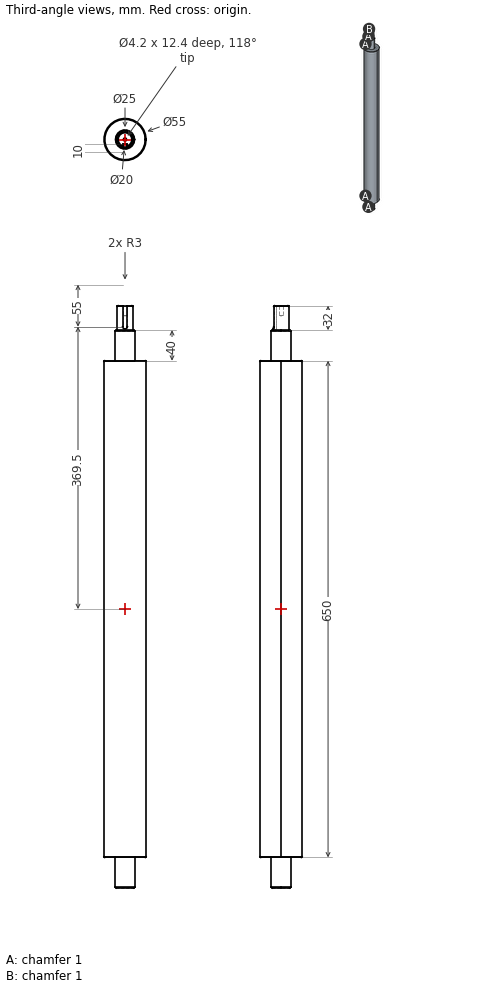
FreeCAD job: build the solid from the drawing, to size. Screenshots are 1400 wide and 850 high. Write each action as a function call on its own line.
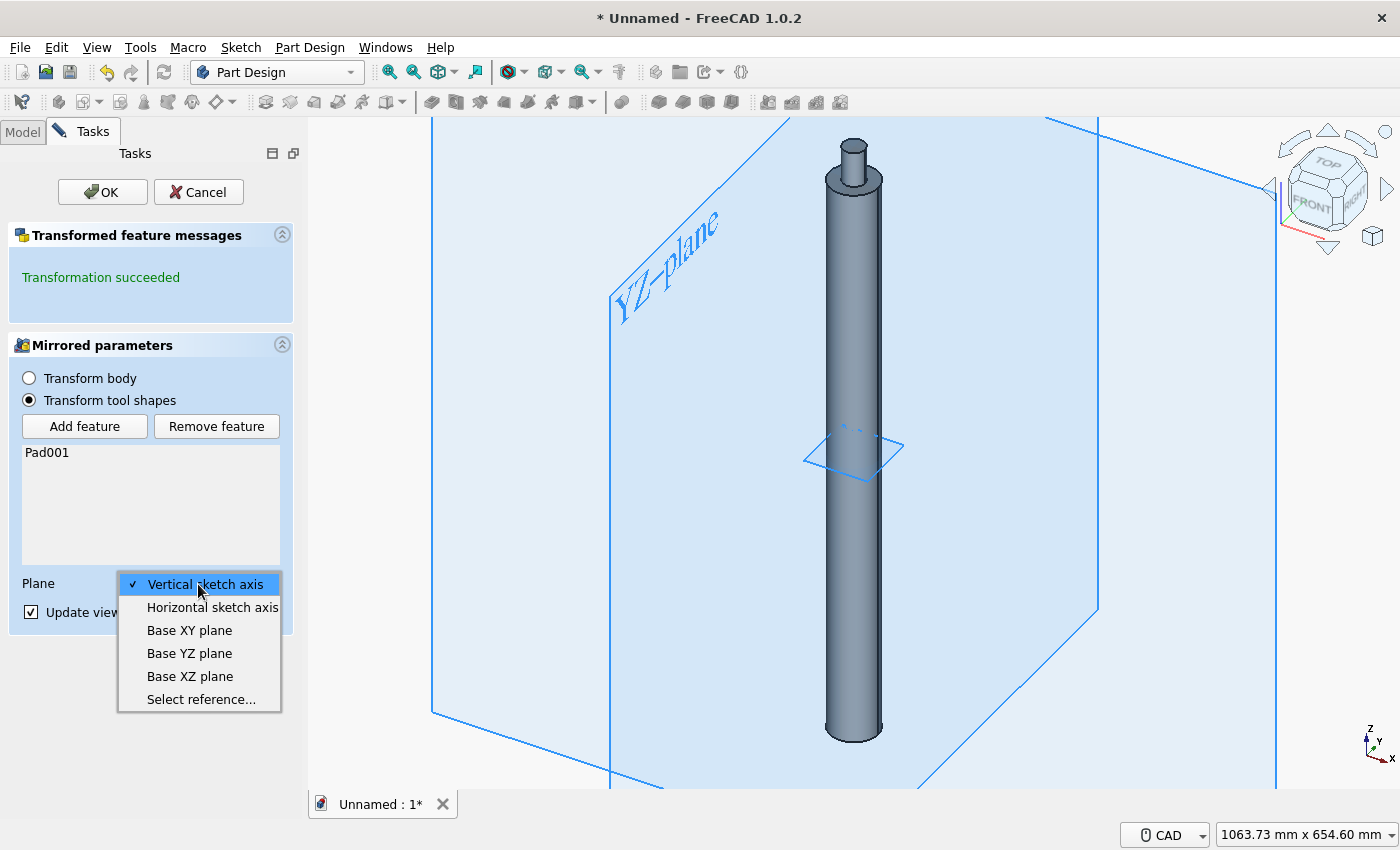
click(198, 630)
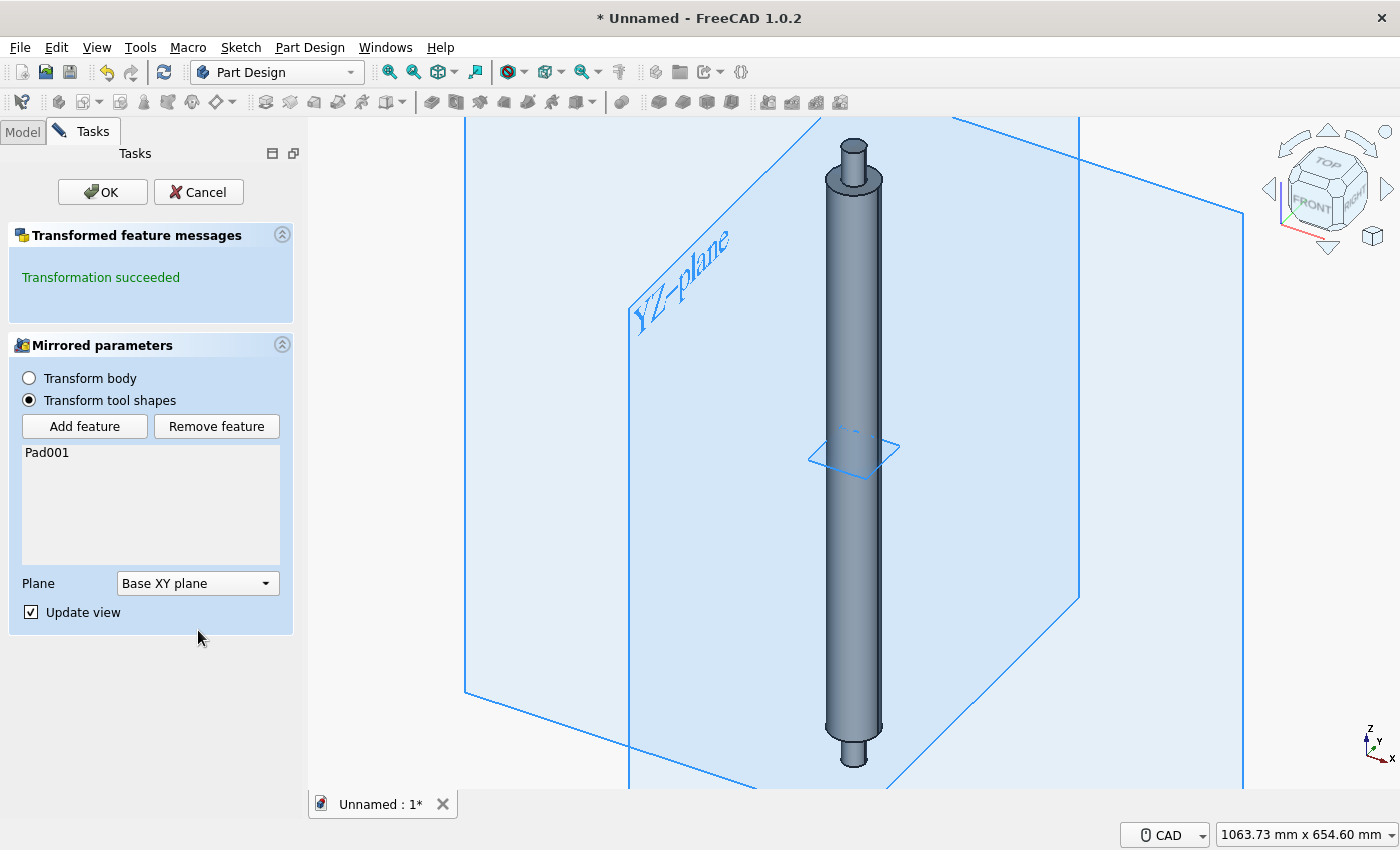
click(103, 192)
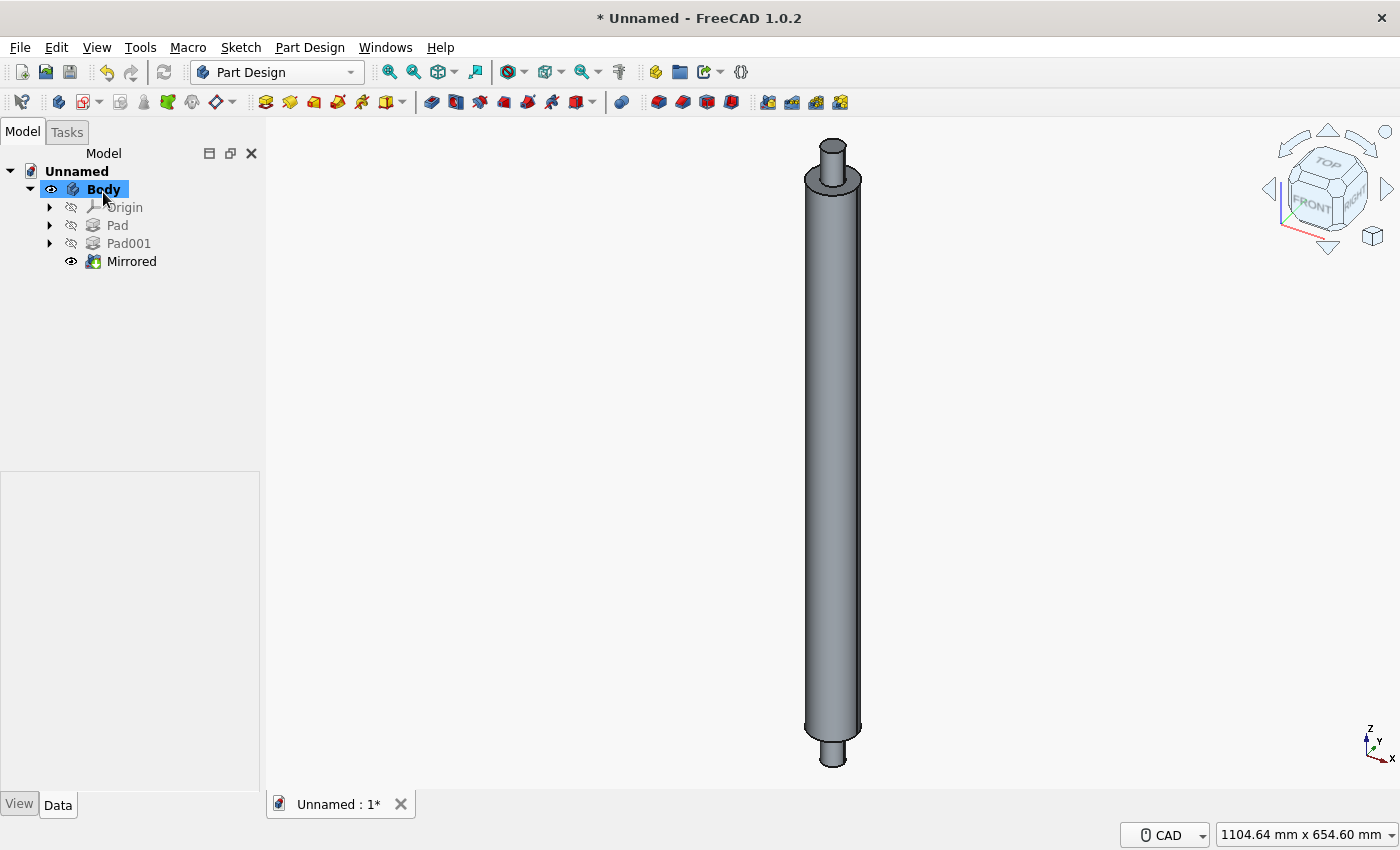
click(805, 180)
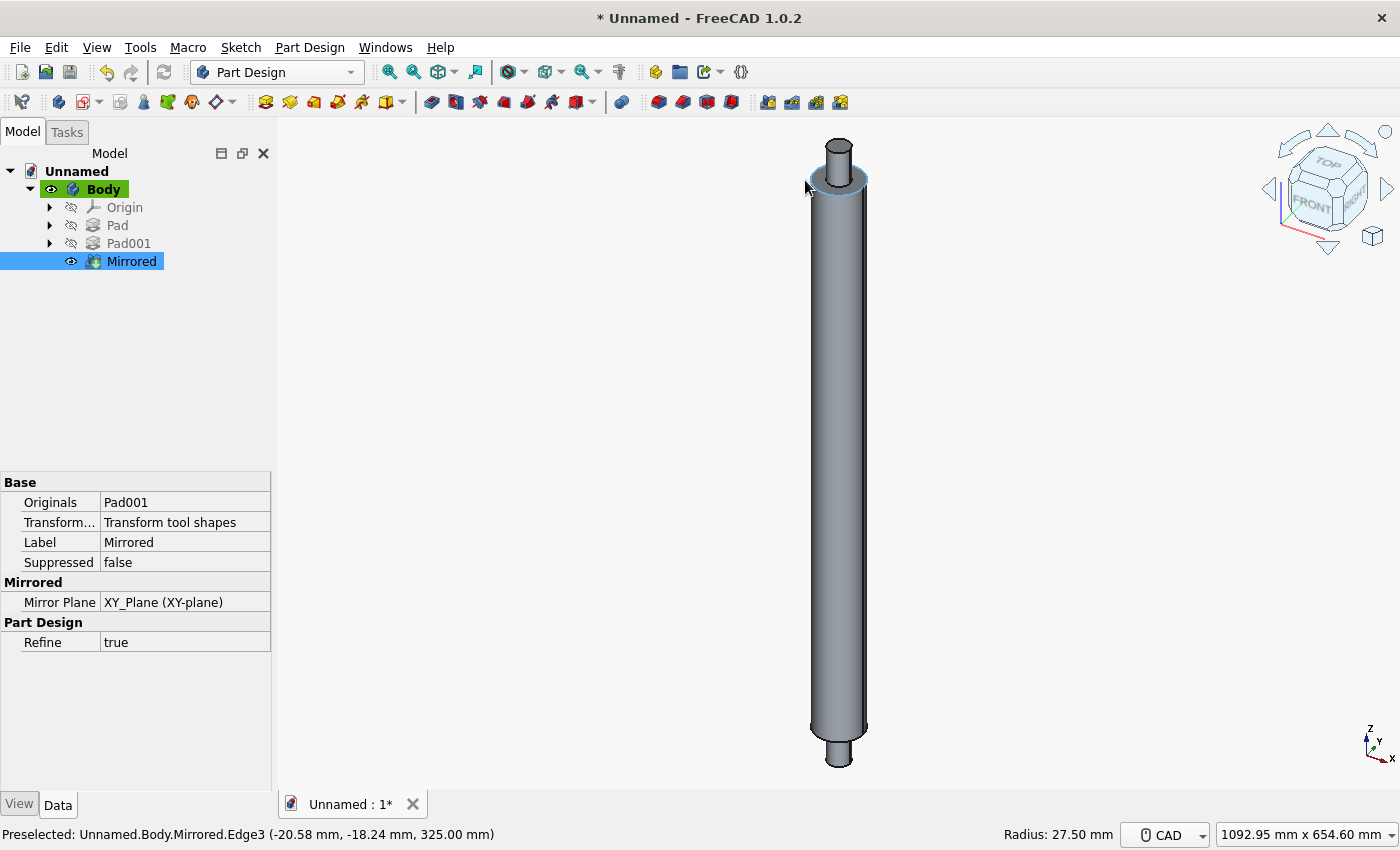
click(826, 146, ctrl)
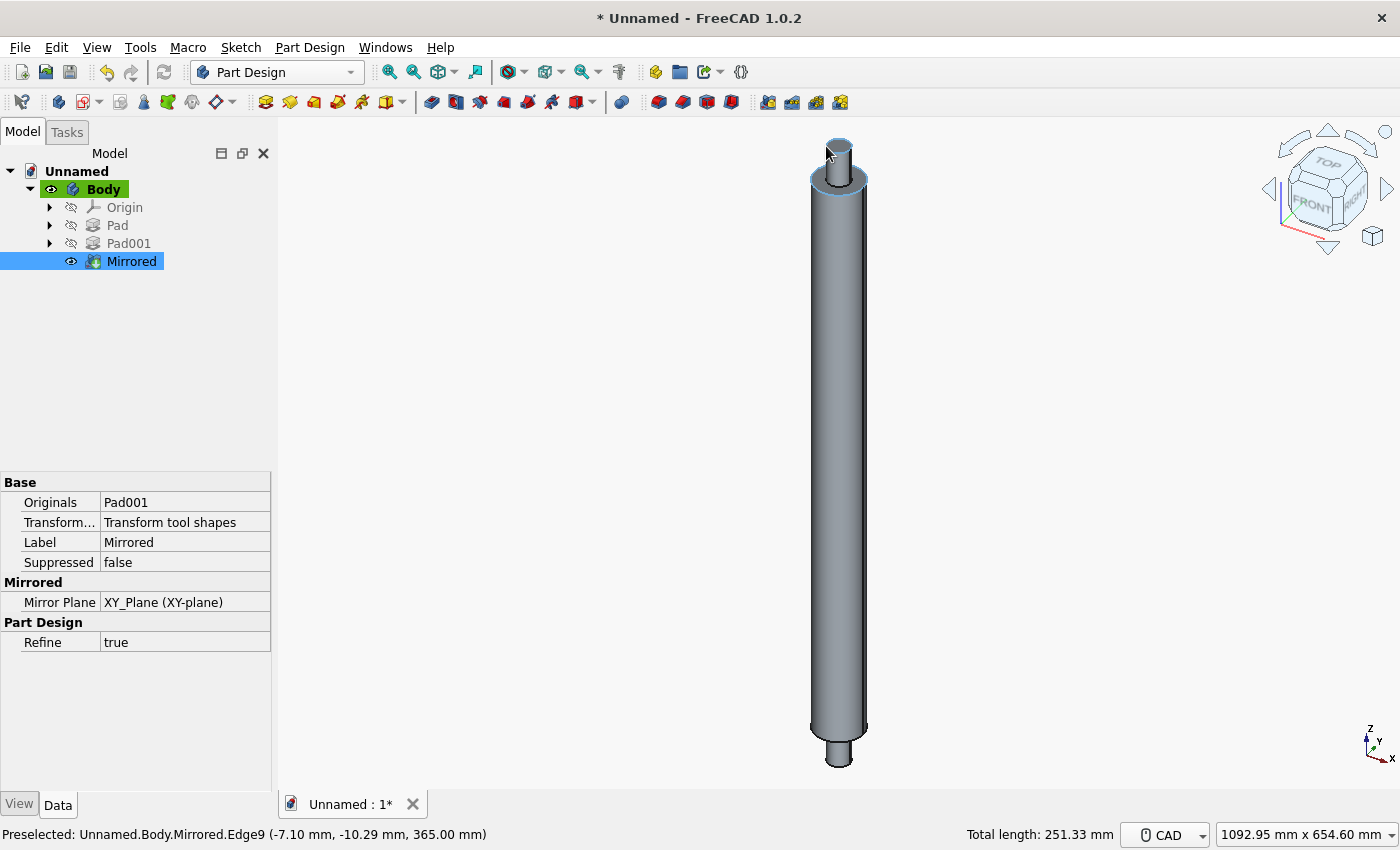
key(0)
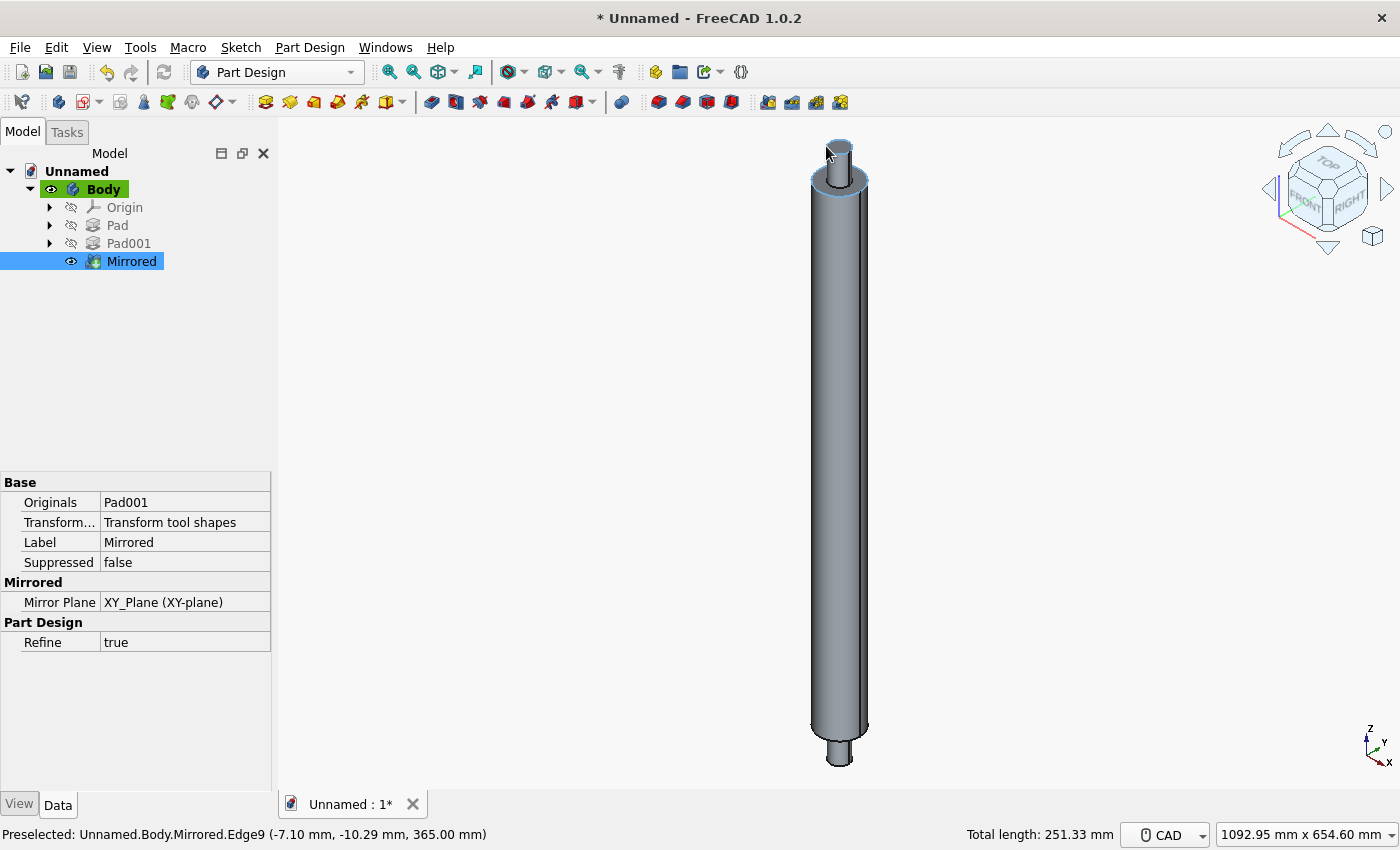
click(814, 732, ctrl)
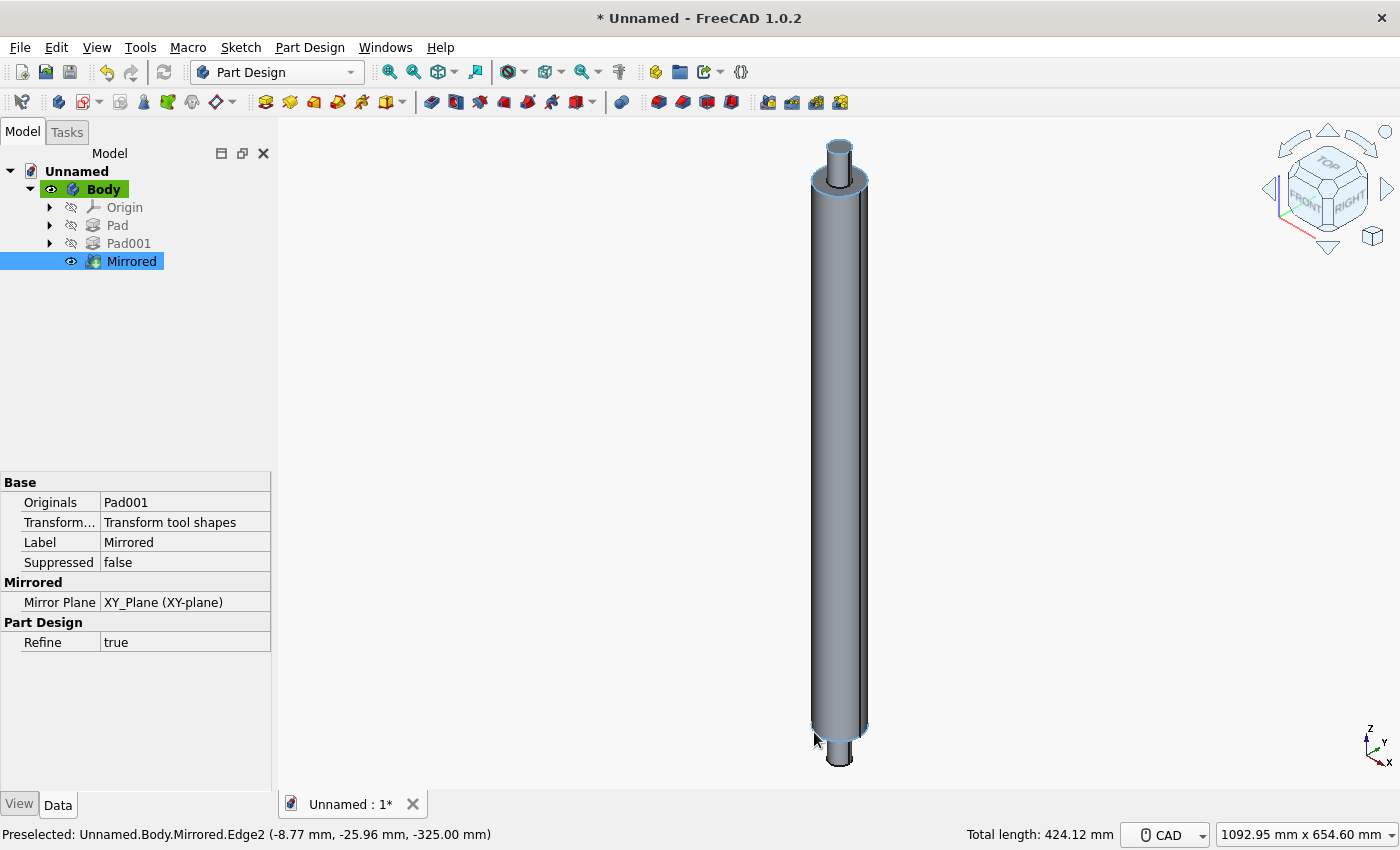
key(2)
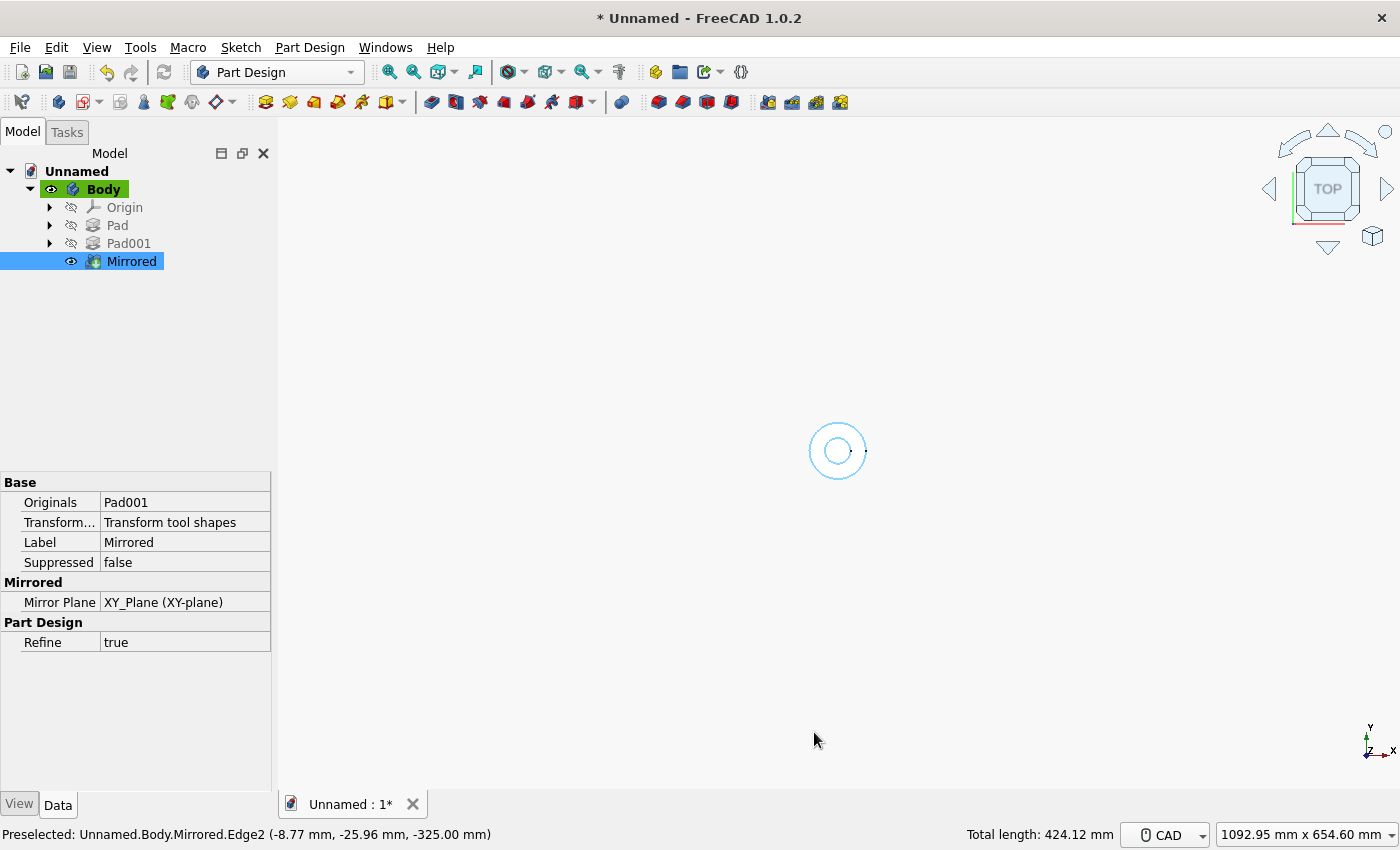
click(390, 72)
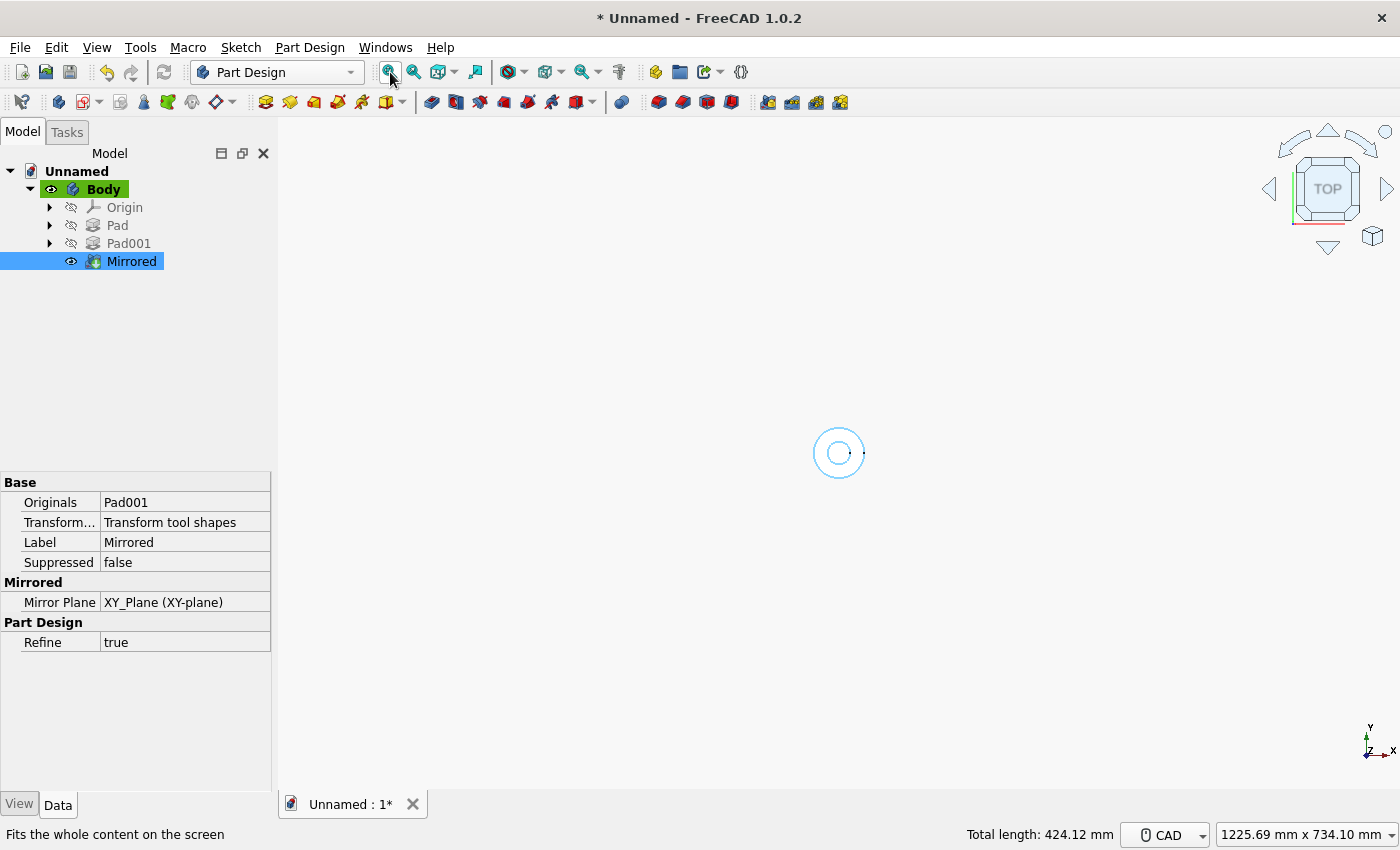
key(1)